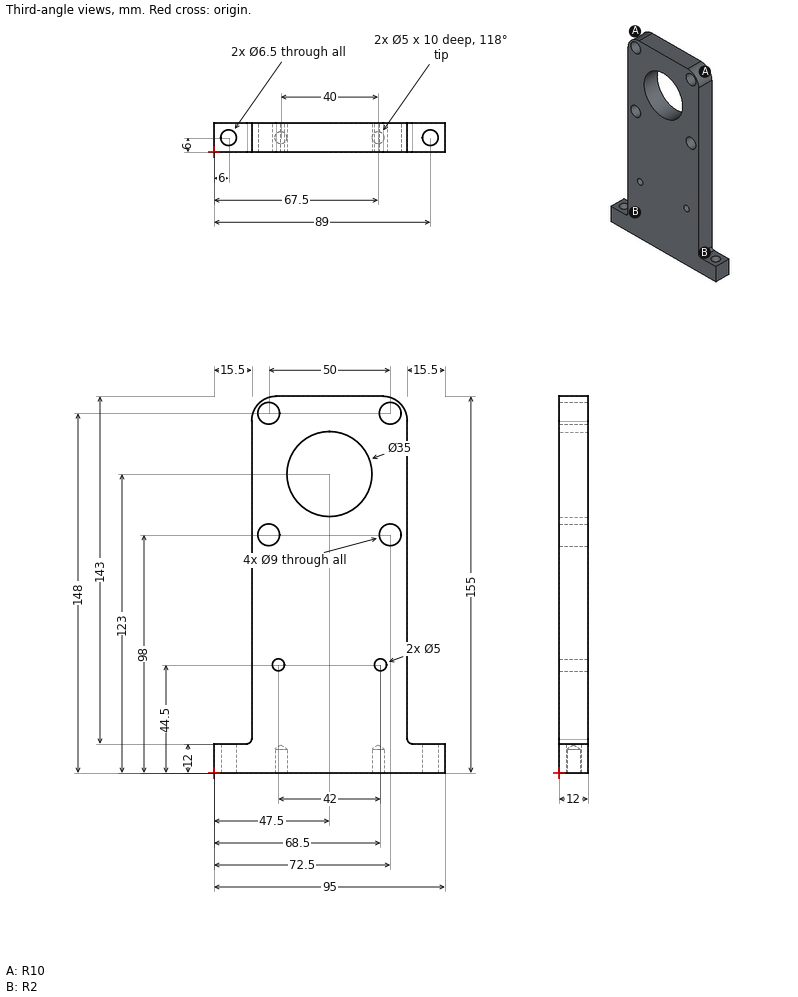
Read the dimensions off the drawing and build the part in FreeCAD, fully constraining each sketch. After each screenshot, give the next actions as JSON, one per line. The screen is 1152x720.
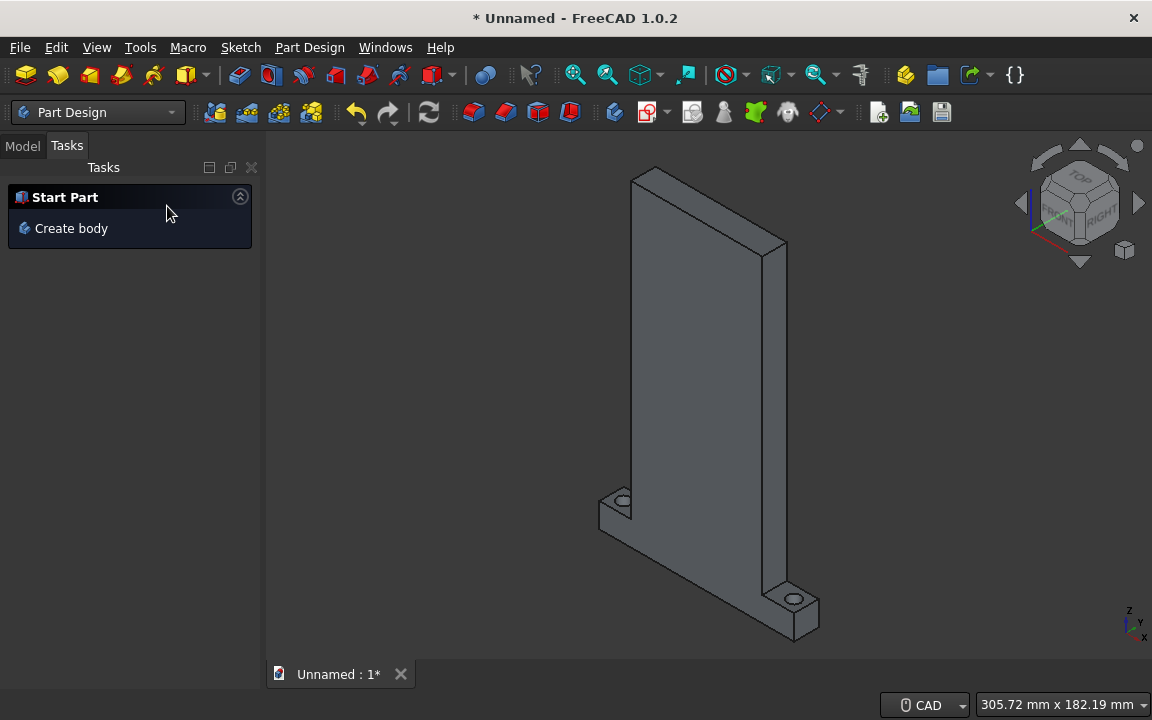
{"action": "key", "text": "4"}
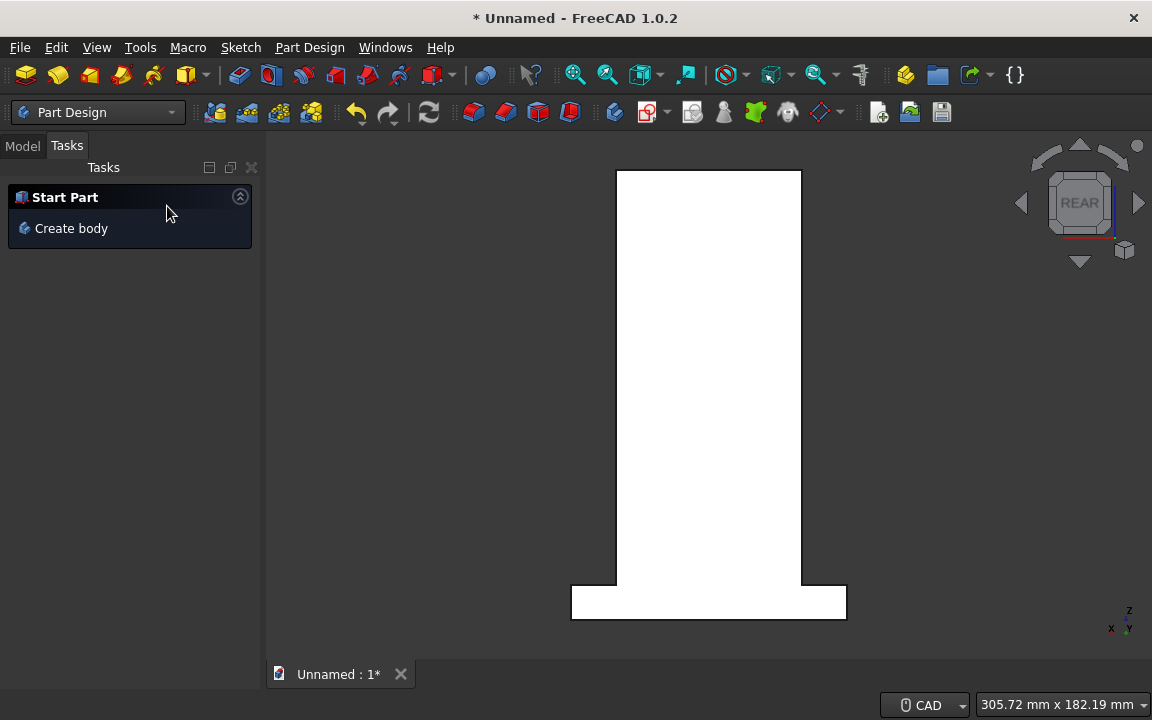
{"action": "left_click", "coordinate": [709, 266]}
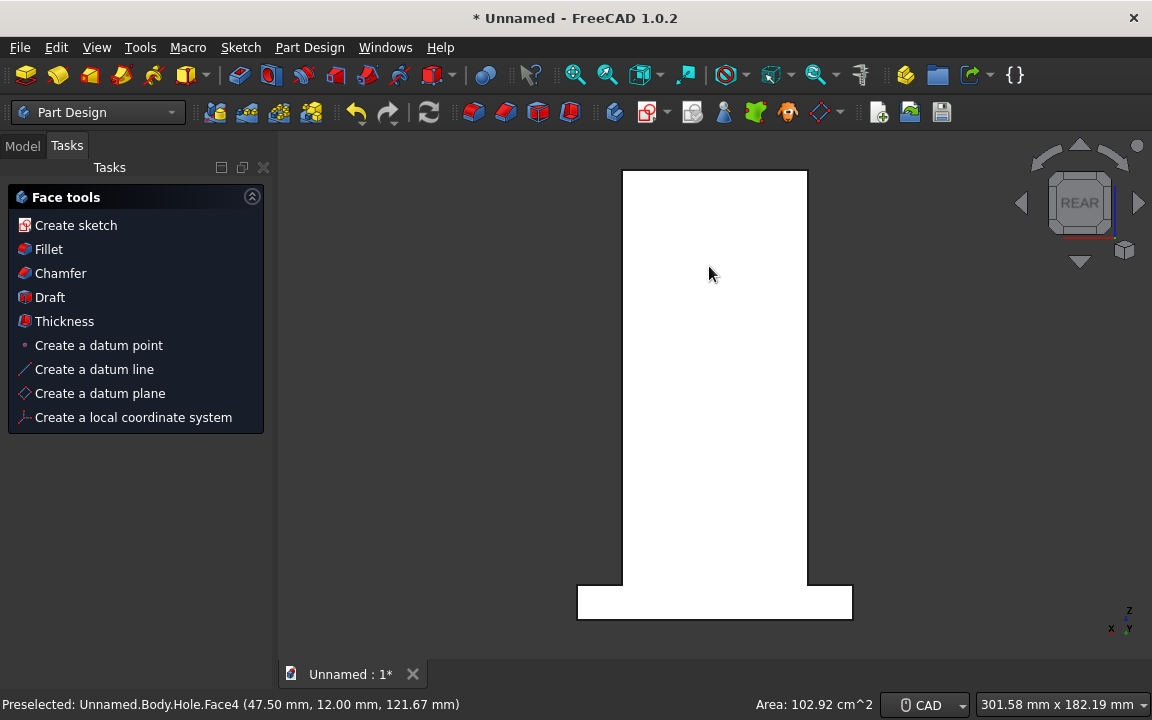
{"action": "left_click", "coordinate": [648, 112]}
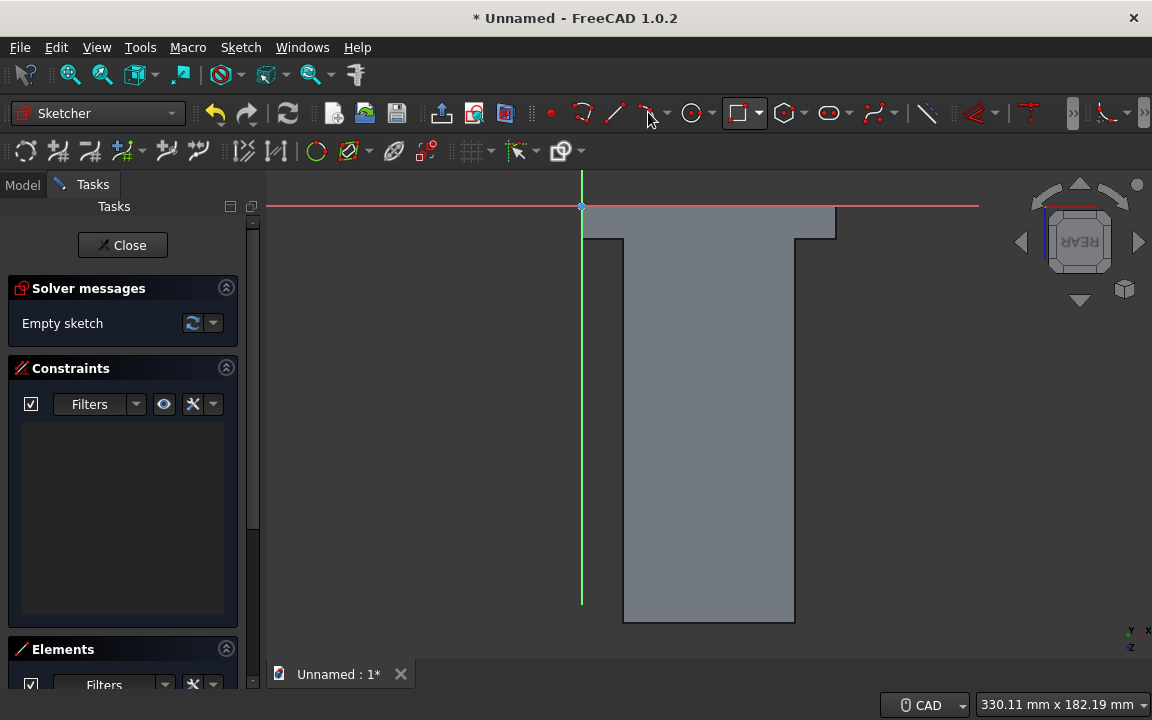
{"action": "scroll", "coordinate": [739, 589], "scroll_direction": "up", "scroll_amount": 6}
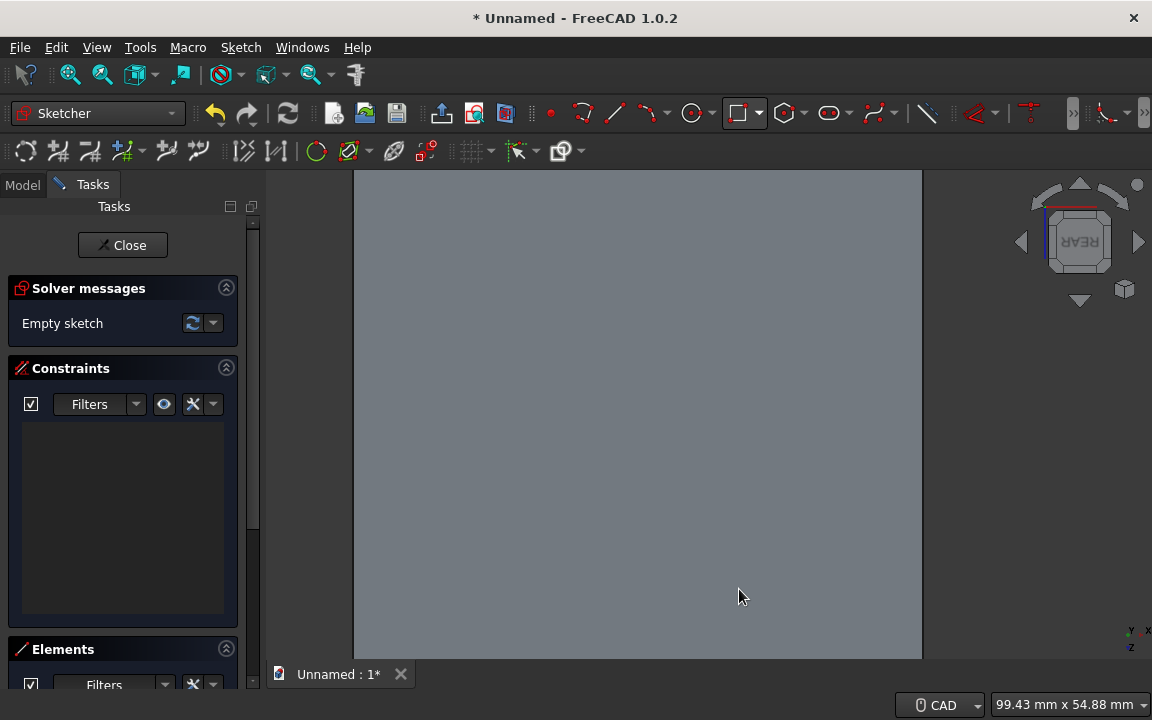
{"action": "left_click", "coordinate": [692, 114]}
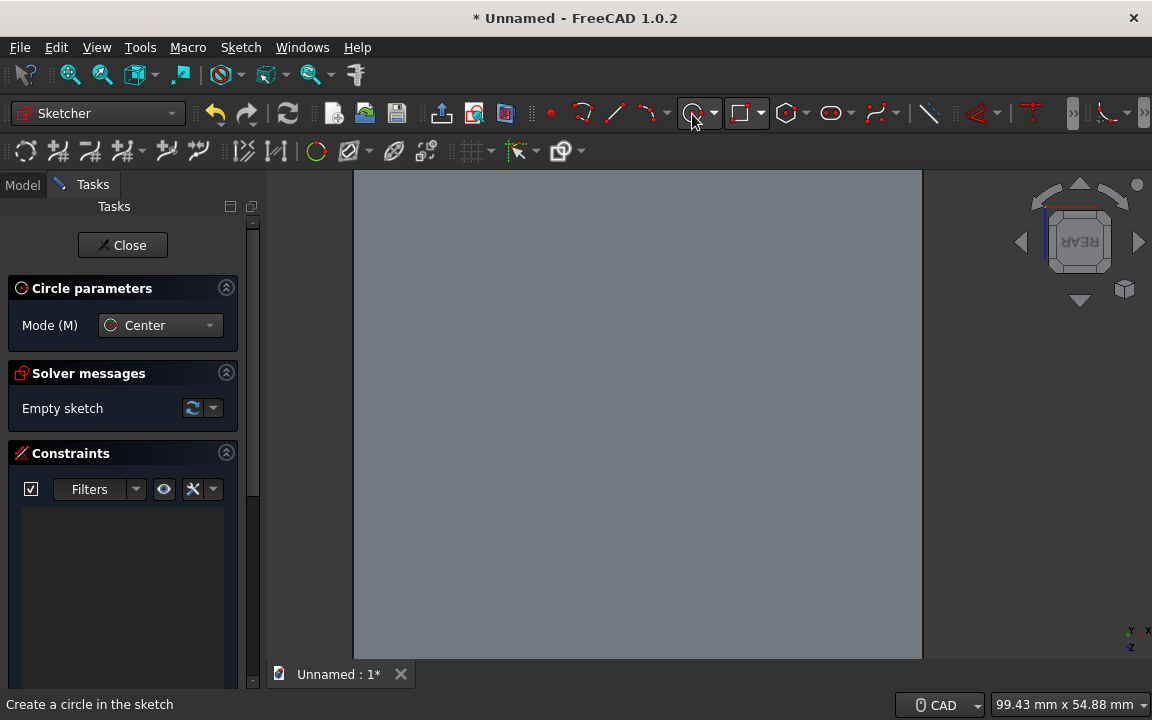
{"action": "left_click", "coordinate": [638, 413]}
{"action": "left_click", "coordinate": [748, 303]}
{"action": "key", "text": "Escape"}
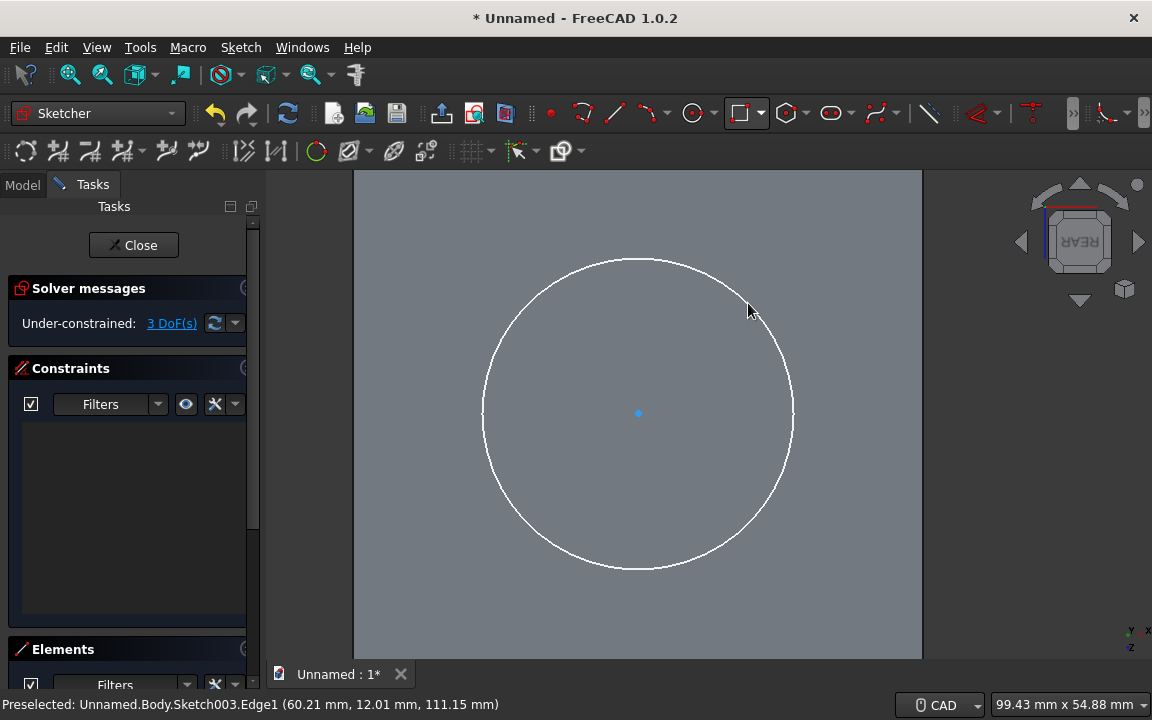
{"action": "left_click", "coordinate": [976, 114]}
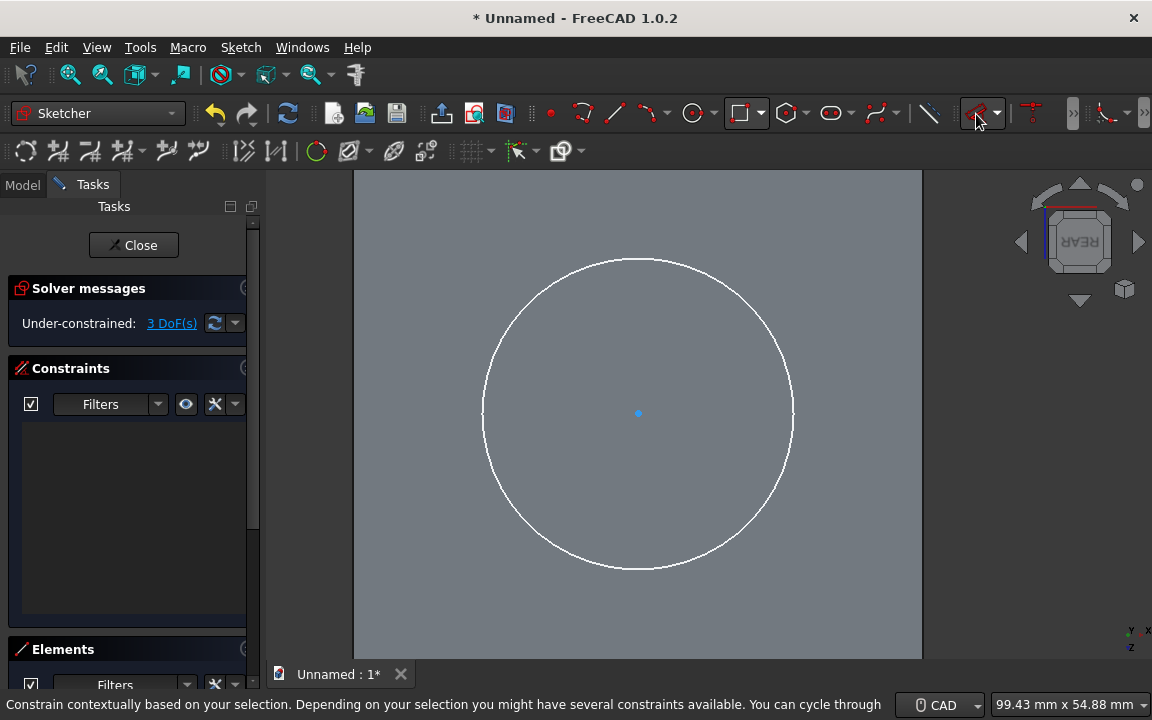
{"action": "left_click", "coordinate": [748, 304]}
{"action": "left_click", "coordinate": [771, 281]}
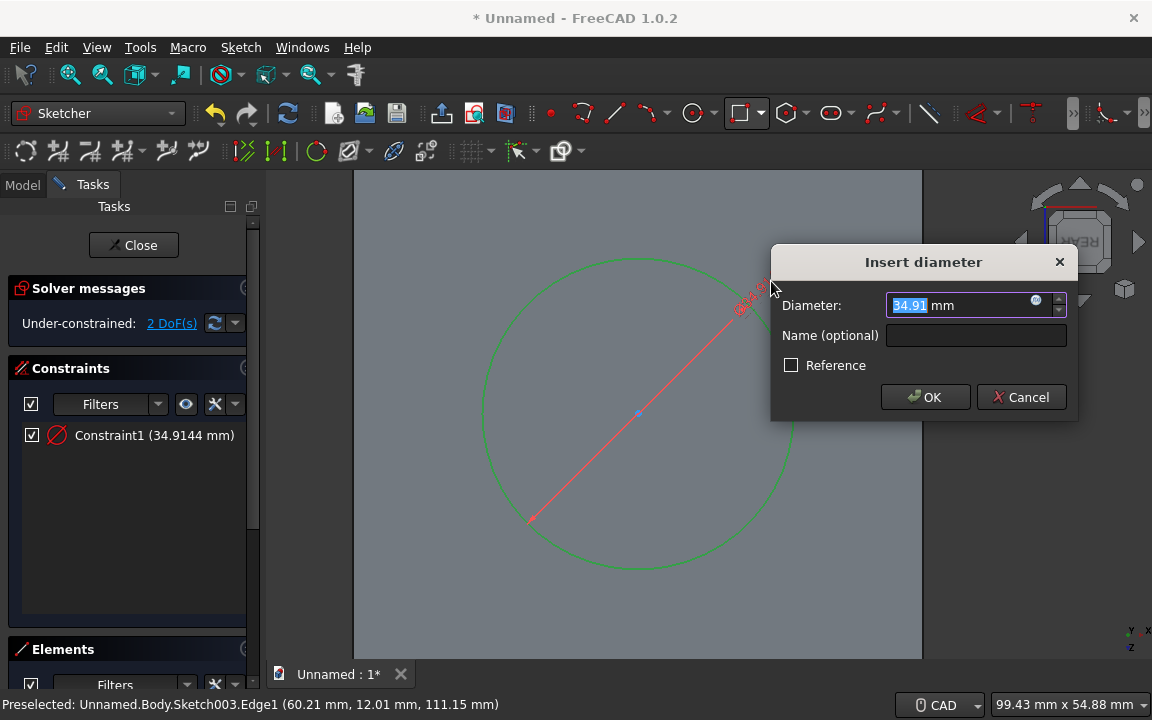
{"action": "type", "text": "35"}
{"action": "key", "text": "Return"}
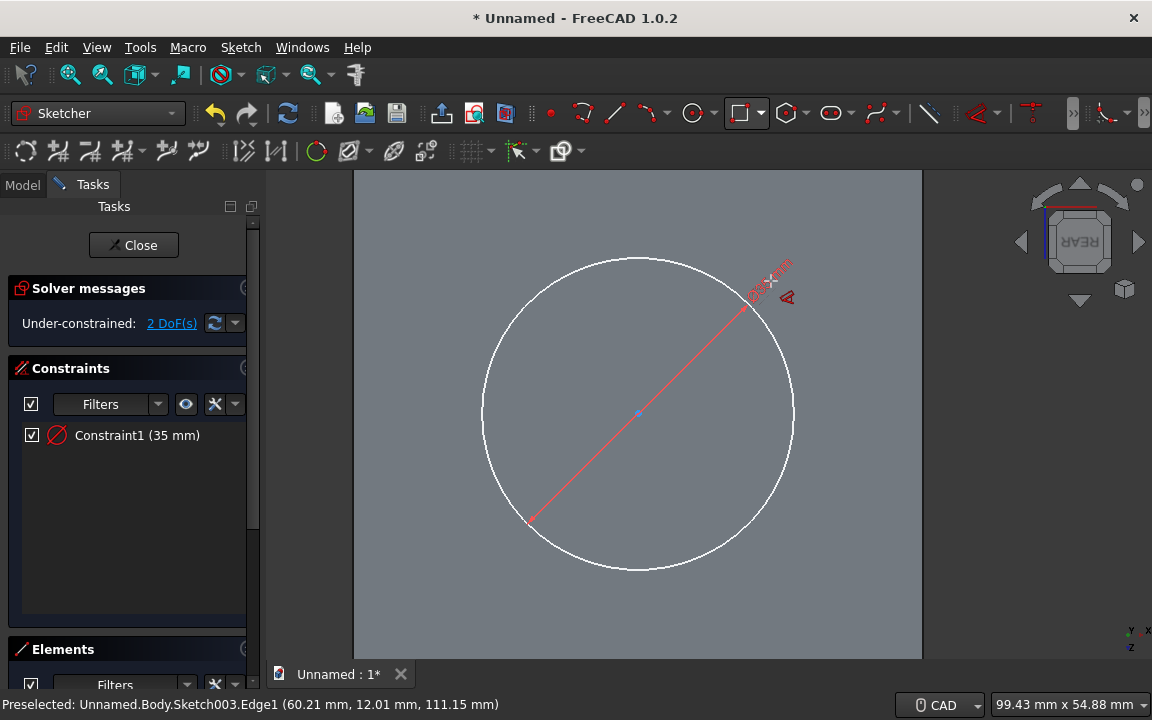
{"action": "left_click", "coordinate": [638, 414]}
{"action": "left_click", "coordinate": [672, 306]}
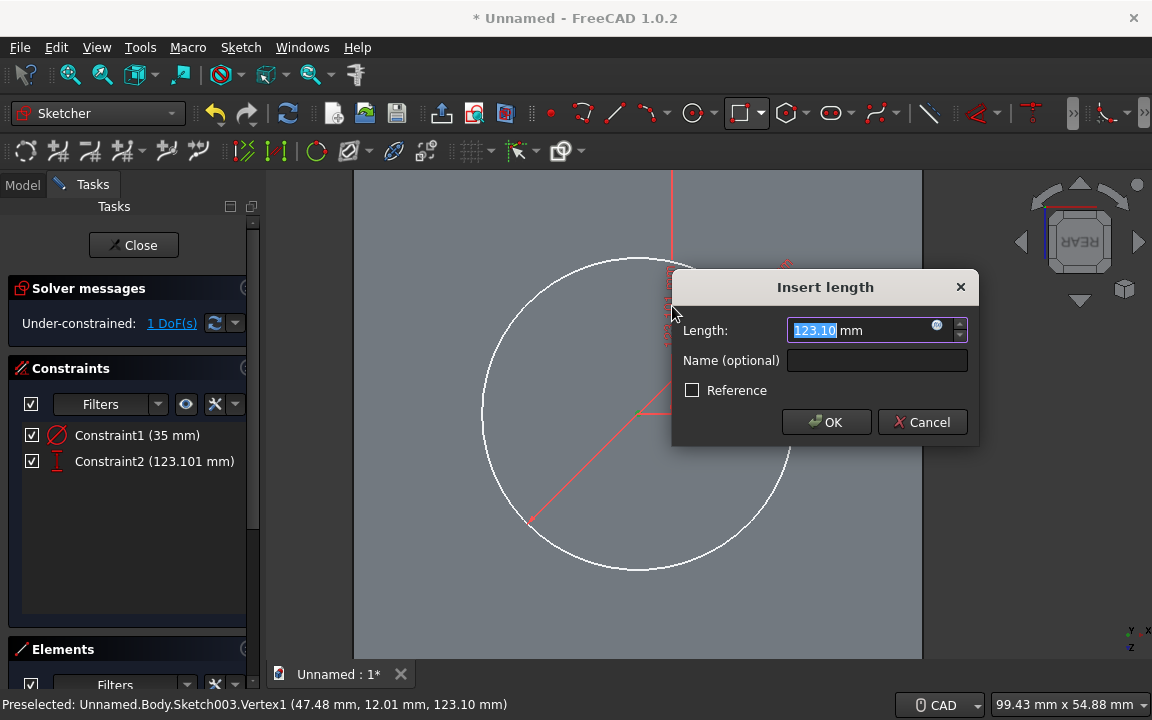
{"action": "type", "text": "123"}
{"action": "key", "text": "Return"}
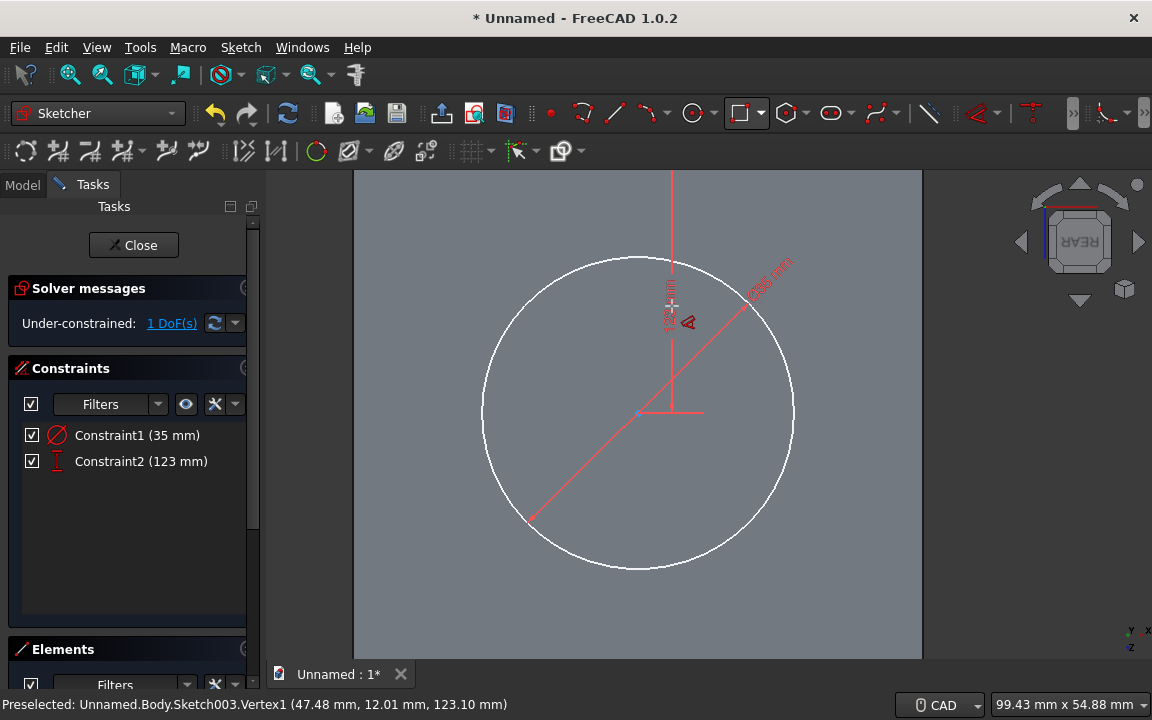
{"action": "left_click", "coordinate": [638, 413]}
{"action": "left_click", "coordinate": [466, 447]}